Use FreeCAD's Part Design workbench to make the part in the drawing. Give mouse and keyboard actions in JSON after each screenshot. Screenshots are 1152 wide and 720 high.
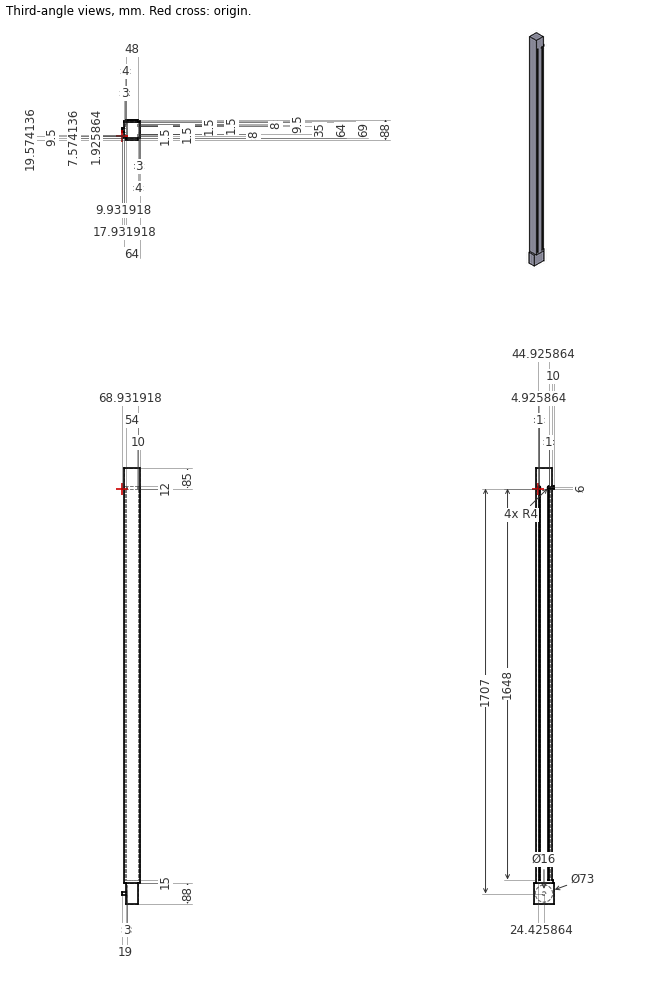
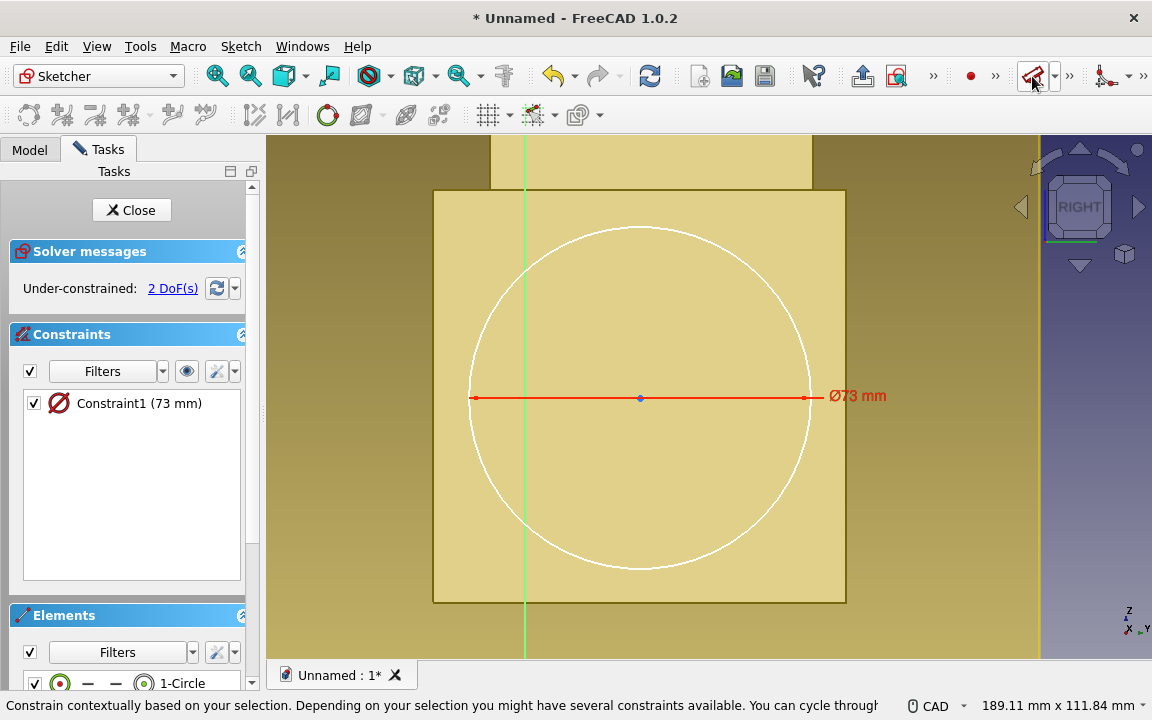
{"action": "left_click", "coordinate": [640, 398]}
{"action": "left_click", "coordinate": [491, 281]}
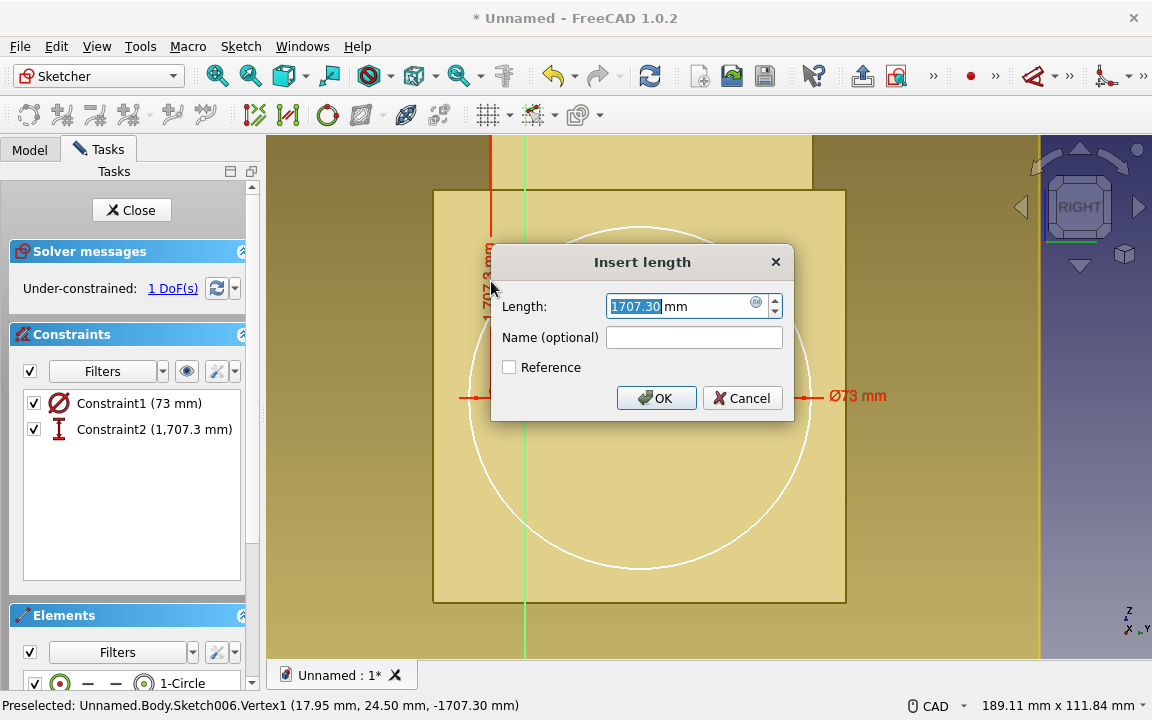
{"action": "type", "text": "1707"}
{"action": "key", "text": "Return"}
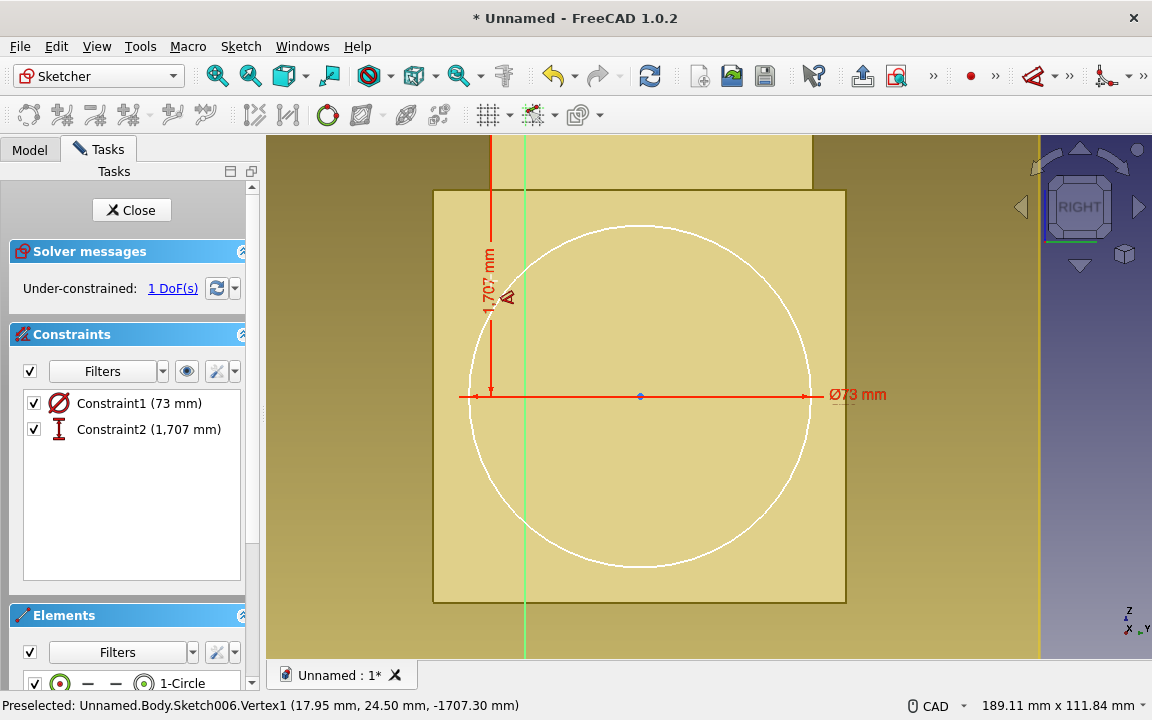
{"action": "left_click", "coordinate": [640, 397]}
{"action": "left_click", "coordinate": [583, 431]}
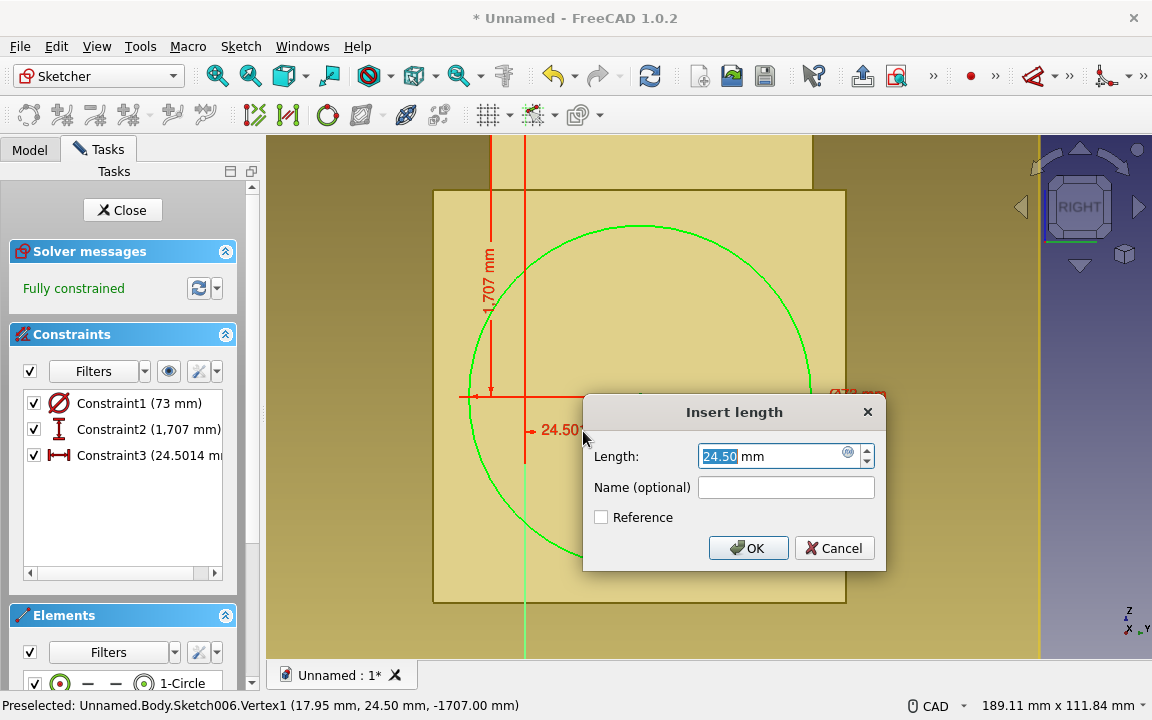
{"action": "type", "text": "24.425864"}
{"action": "key", "text": "Return"}
{"action": "key", "text": "Escape"}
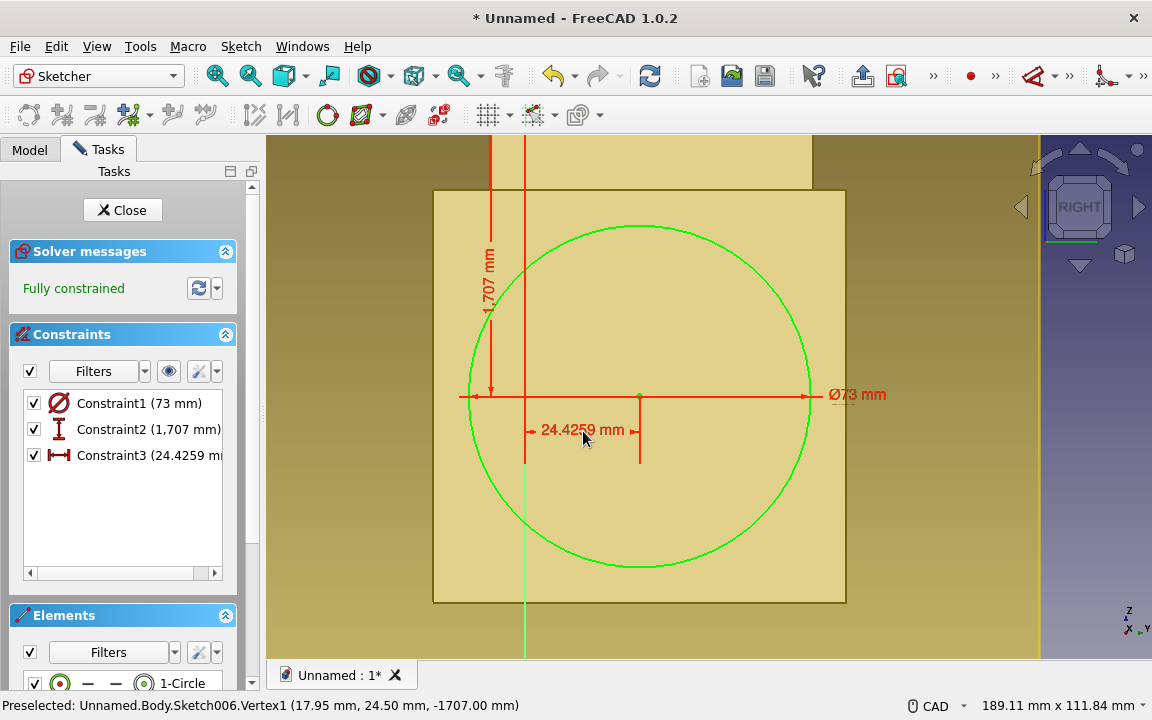
{"action": "left_click", "coordinate": [123, 210]}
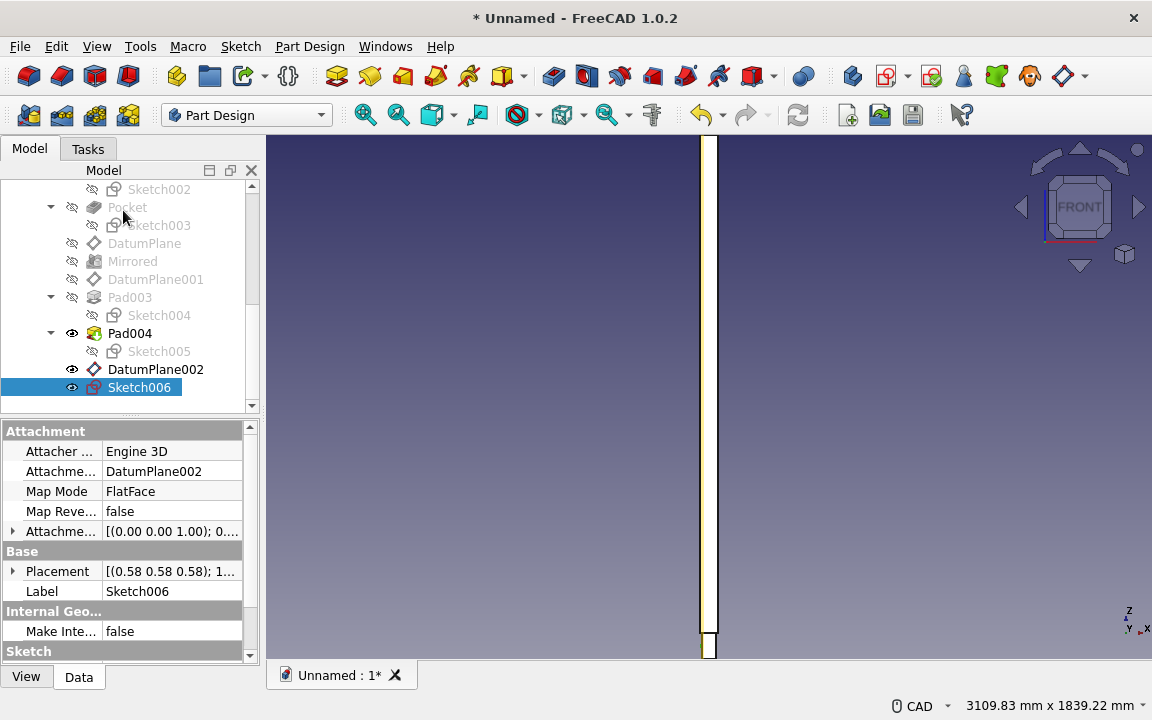
{"action": "left_click", "coordinate": [554, 76]}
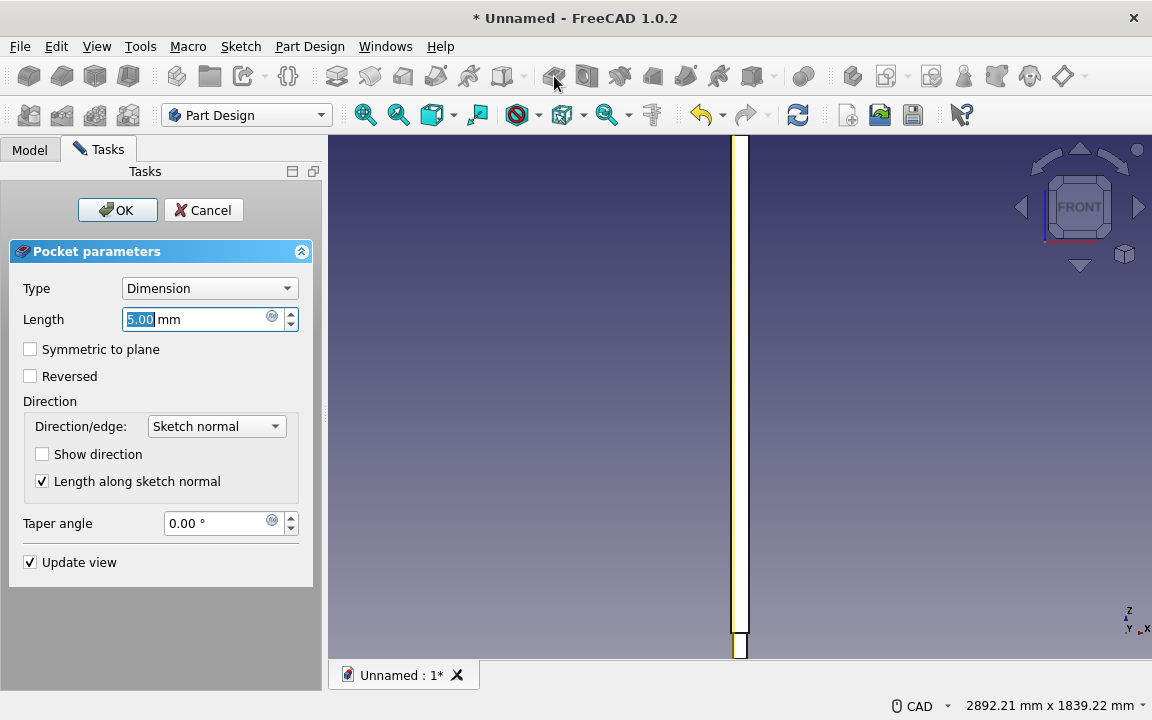
{"action": "type", "text": "3"}
{"action": "key", "text": "Tab"}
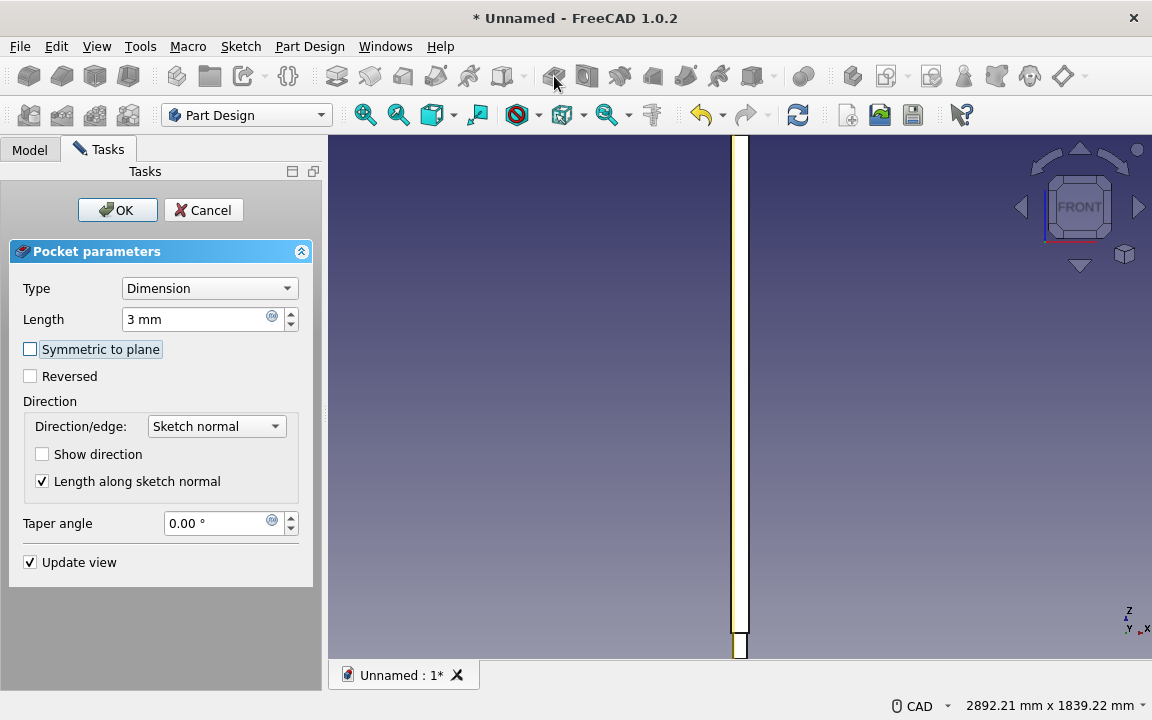
{"action": "left_click", "coordinate": [31, 376]}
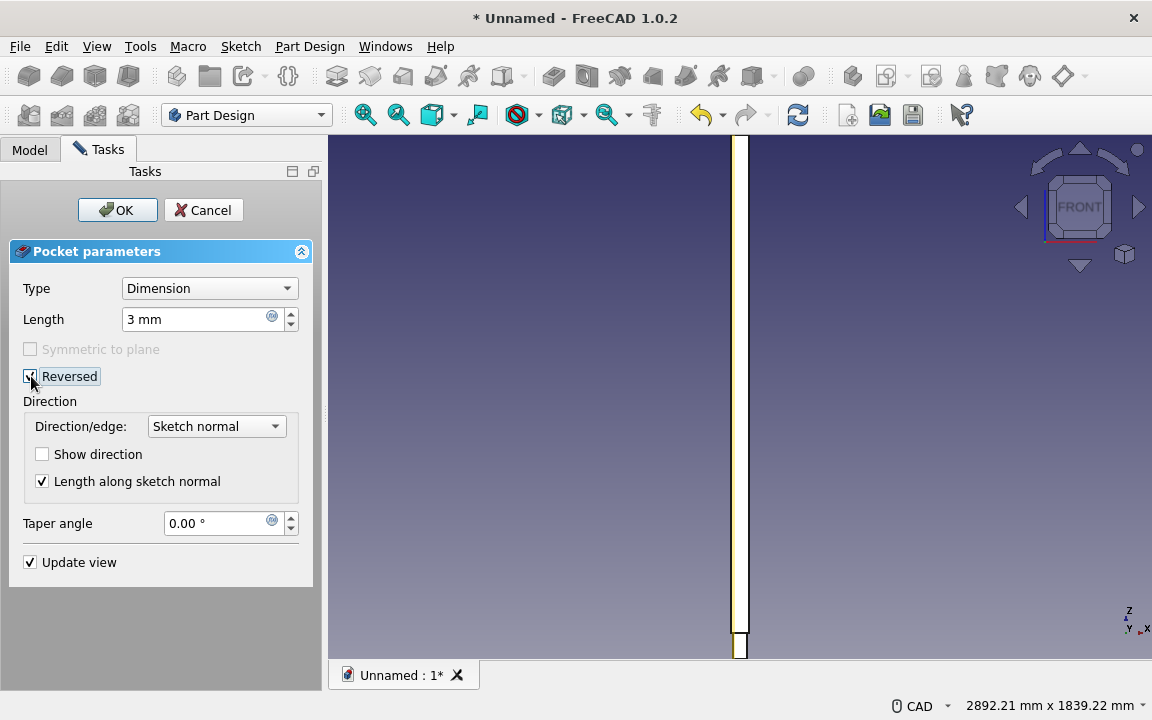
{"action": "left_click", "coordinate": [118, 210]}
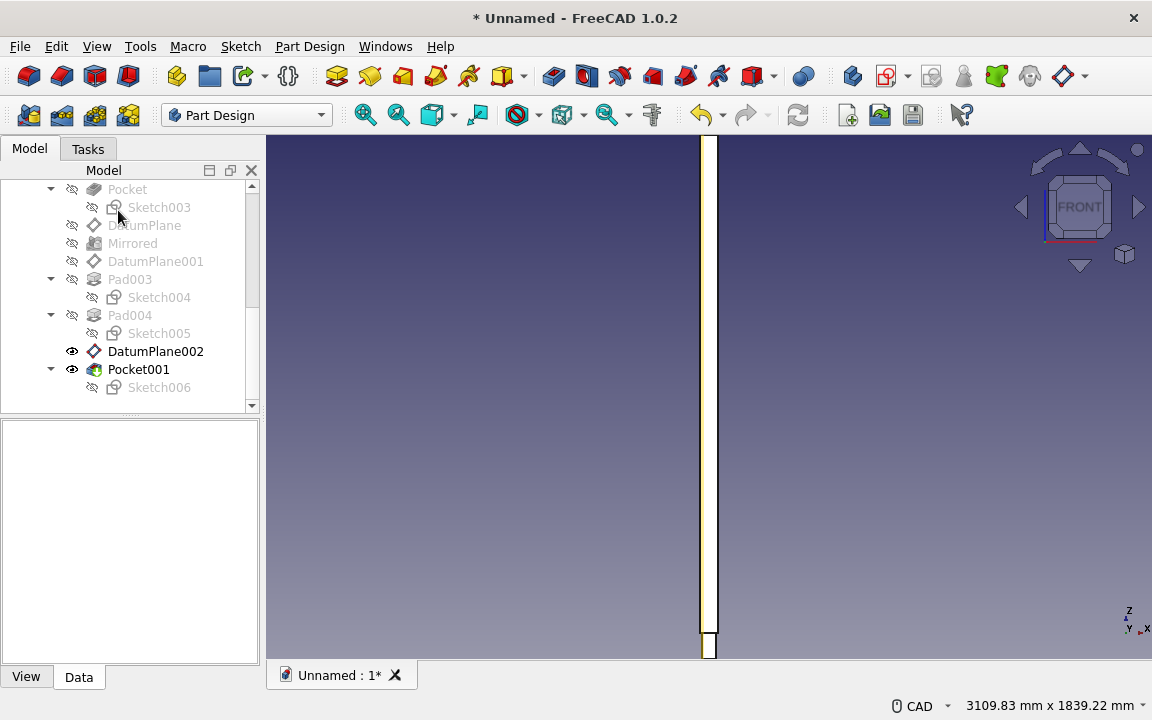
{"action": "left_click", "coordinate": [117, 351]}
{"action": "key", "text": "space"}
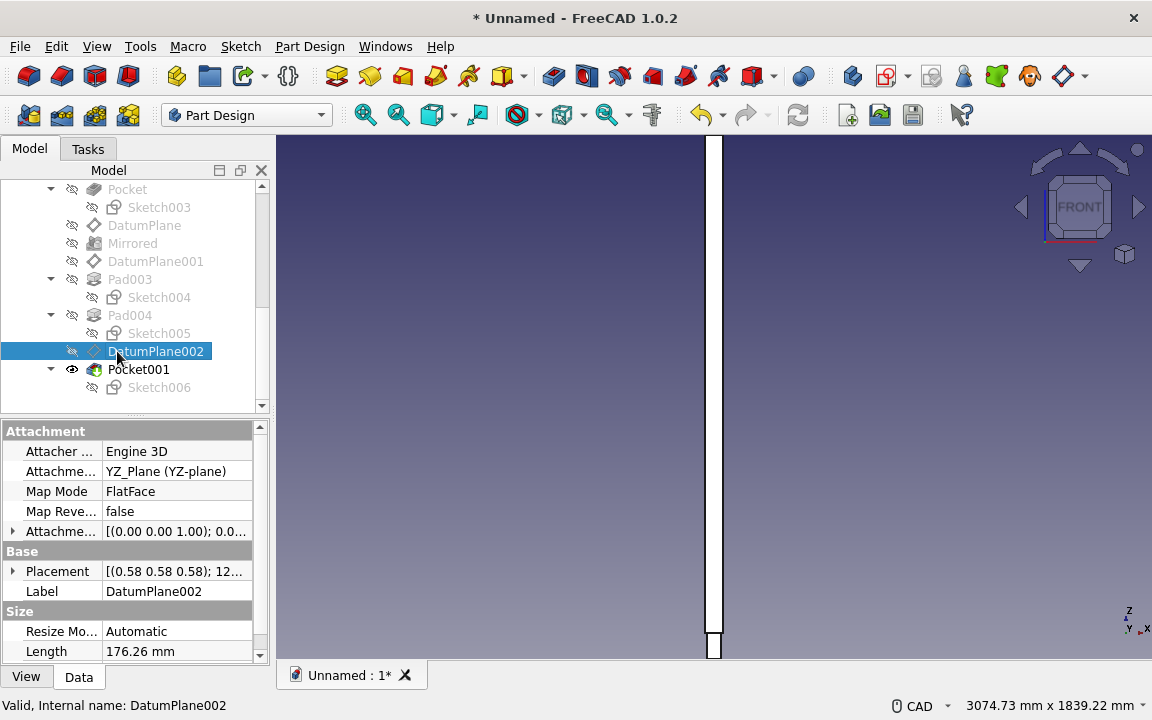
{"action": "left_click", "coordinate": [366, 116]}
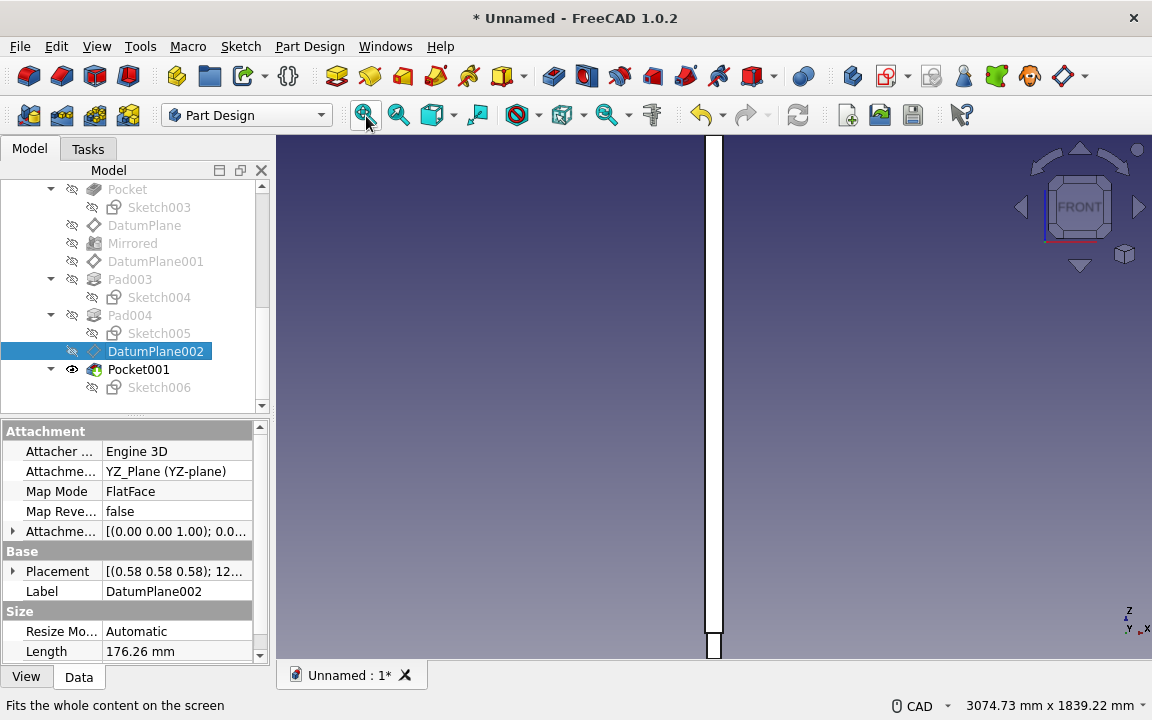
{"action": "key", "text": "6"}